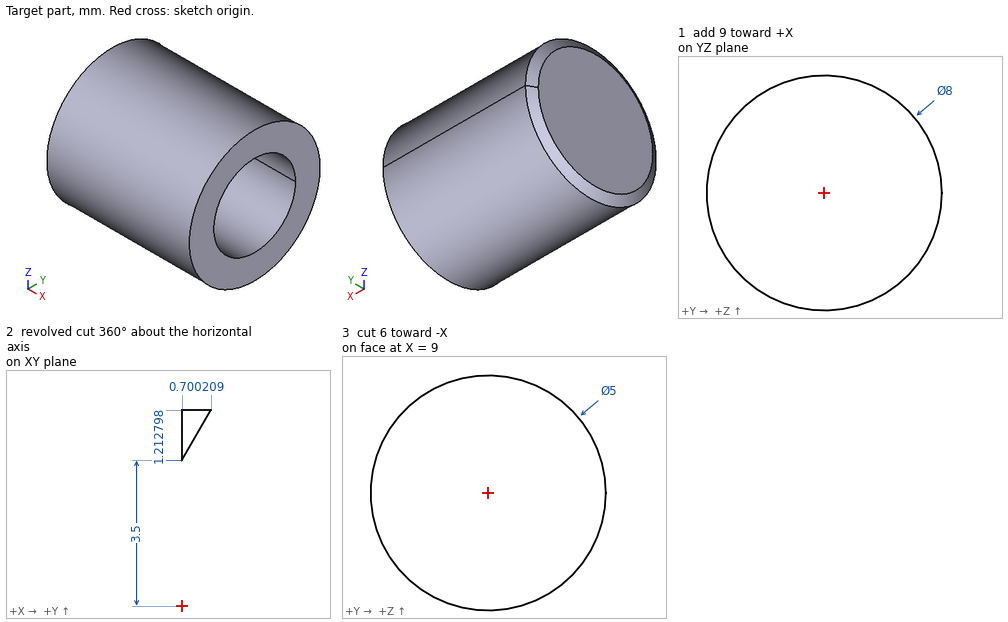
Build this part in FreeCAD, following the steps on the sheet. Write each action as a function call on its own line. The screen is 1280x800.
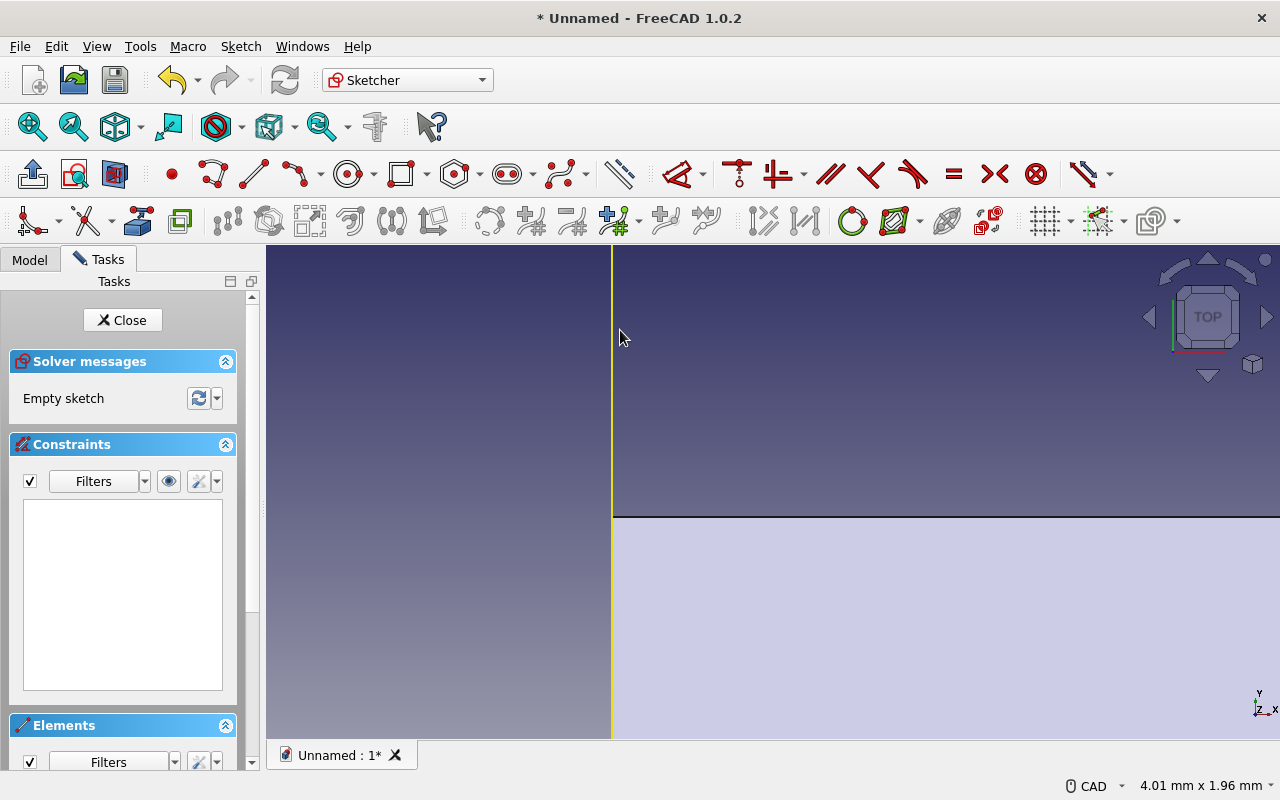
click(213, 174)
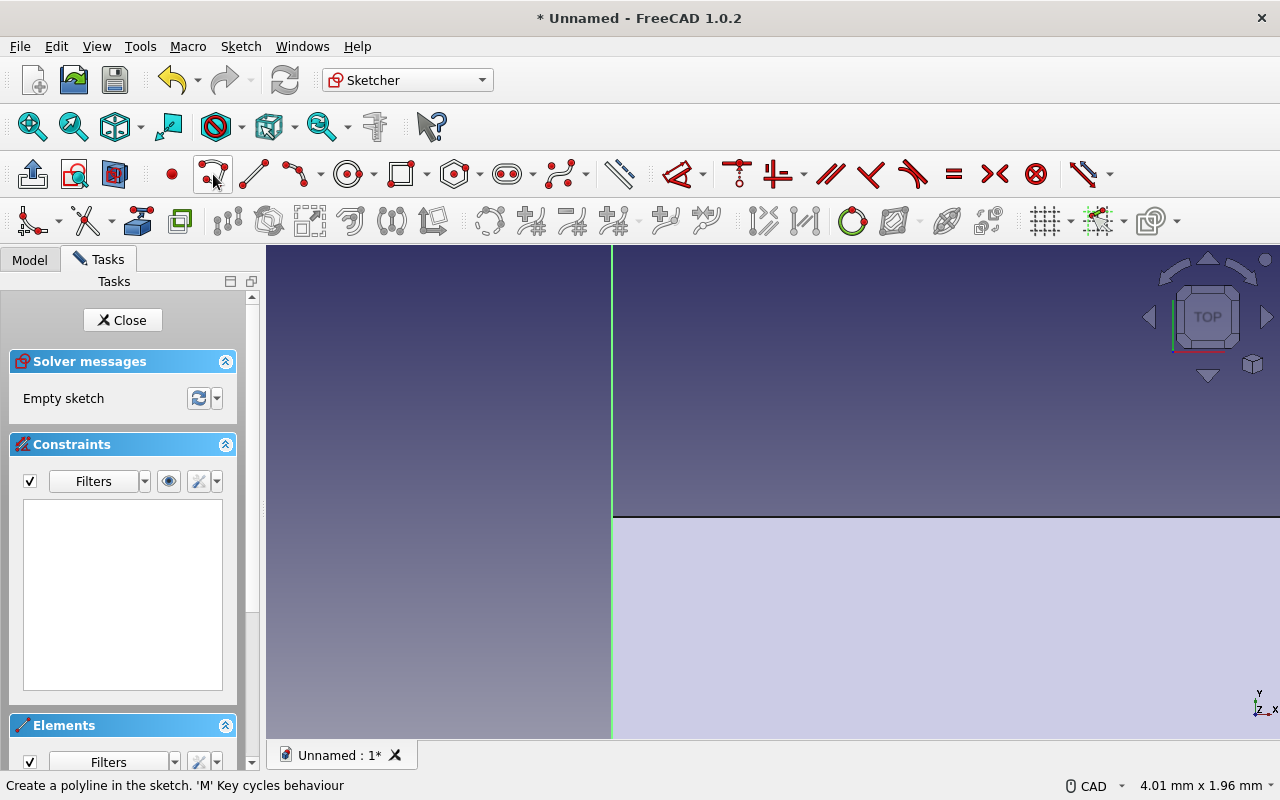
click(612, 643)
click(788, 336)
click(621, 336)
click(612, 644)
key(Escape)
key(Escape)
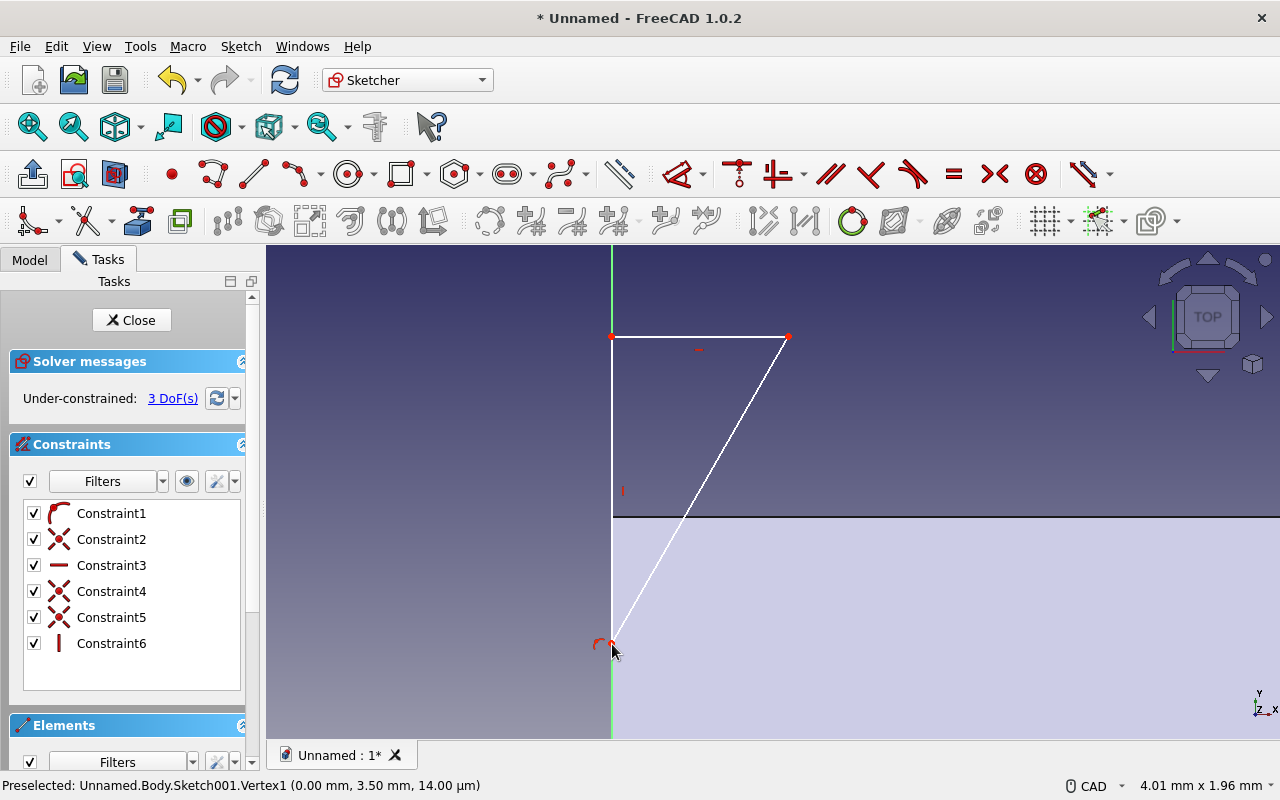
click(676, 174)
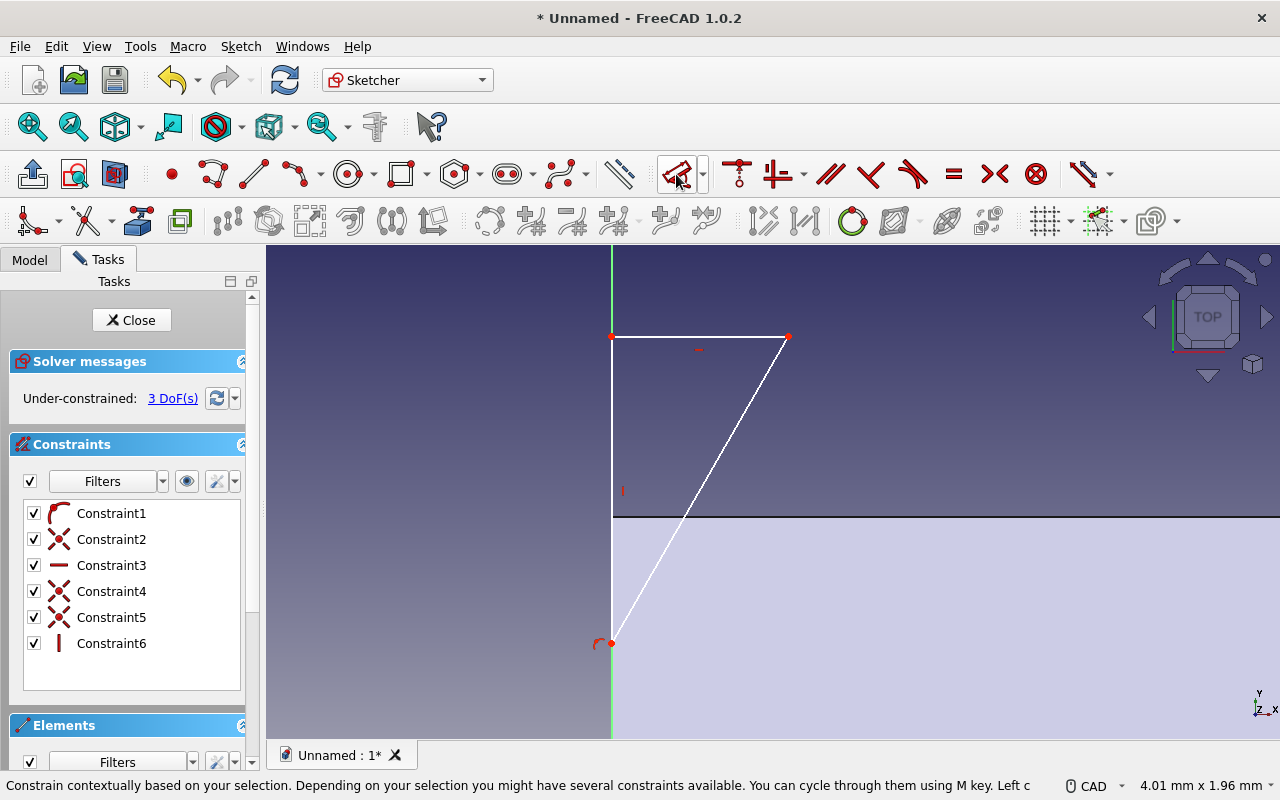
click(612, 644)
click(578, 677)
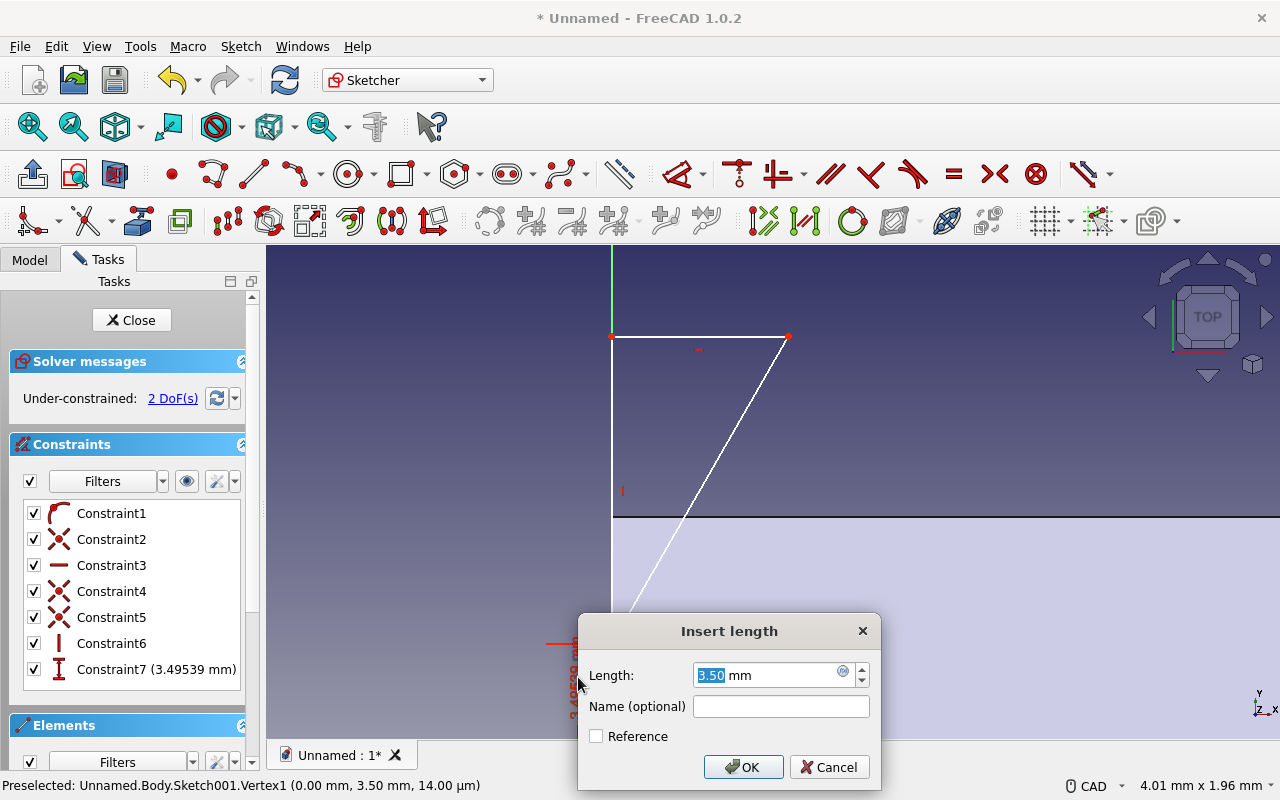
text(3.5)
key(Return)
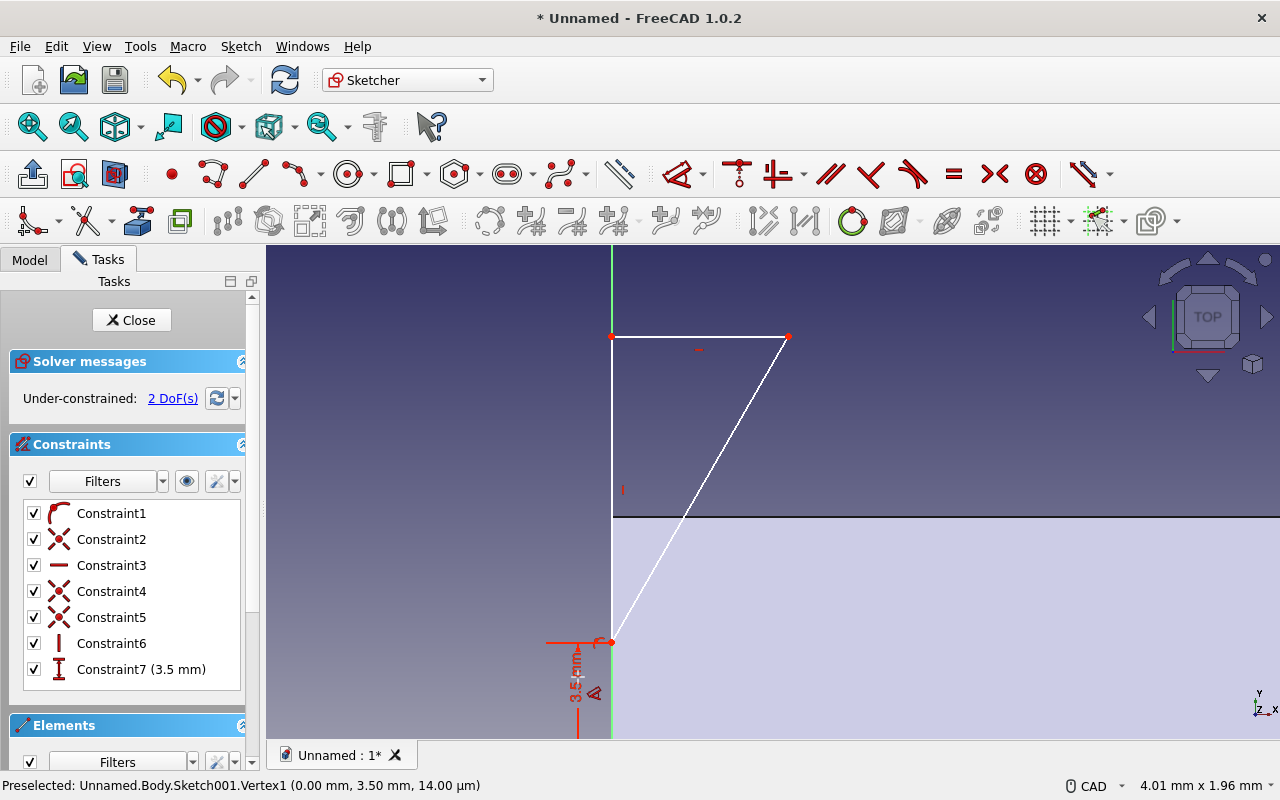
click(735, 337)
click(700, 303)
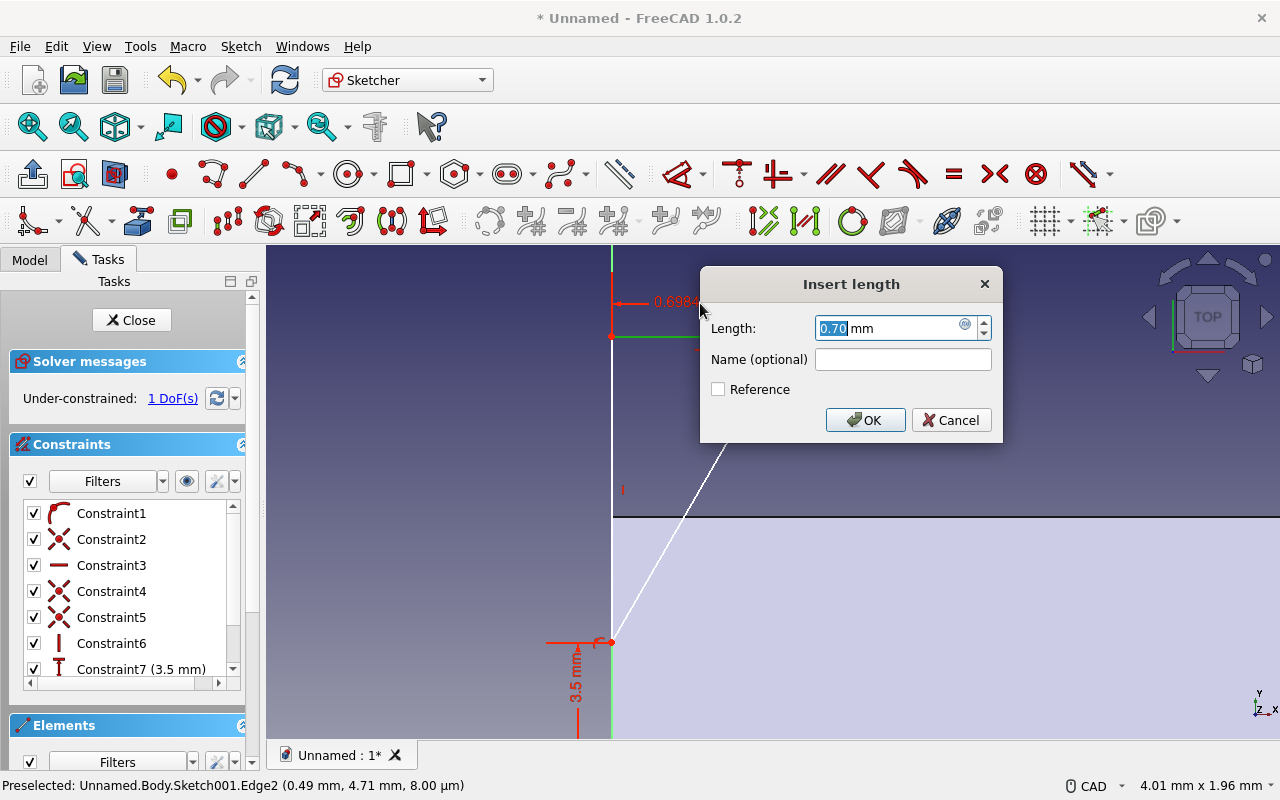
text(0.700209)
key(Return)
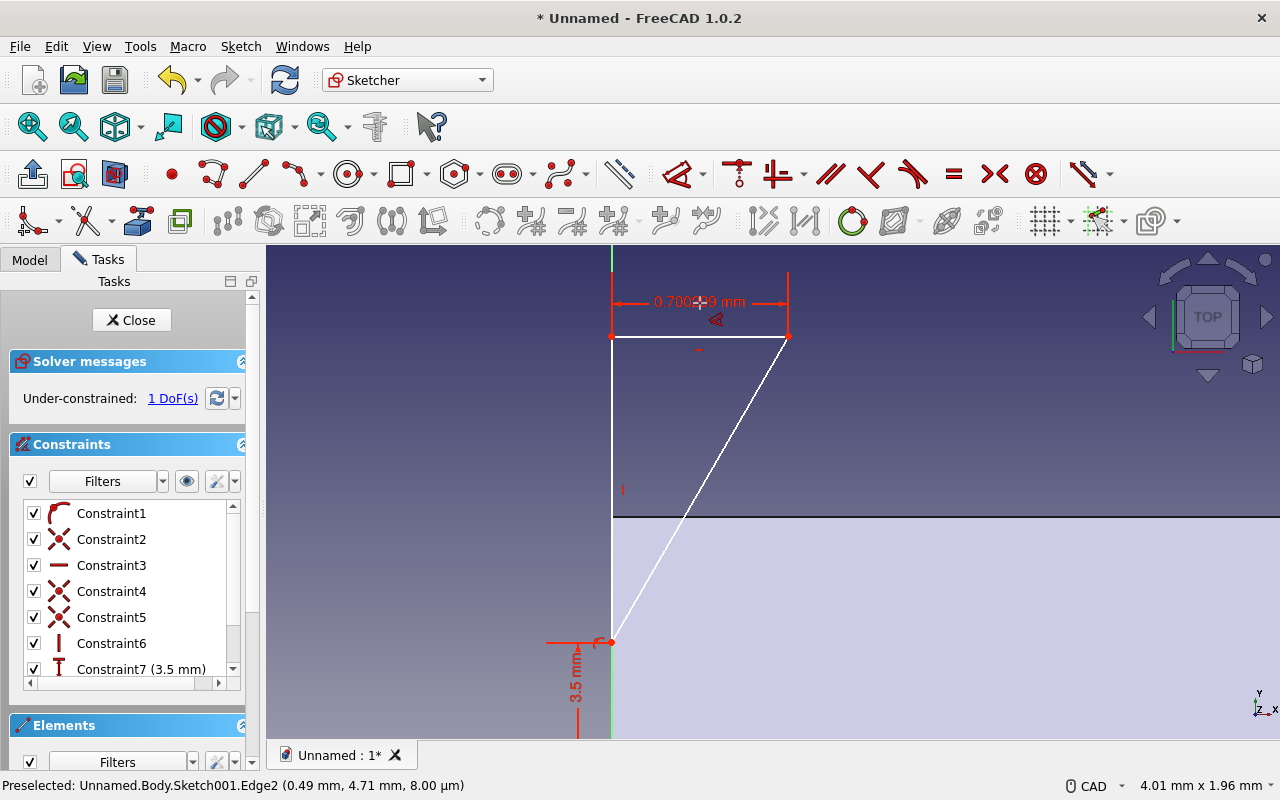
click(612, 429)
click(578, 490)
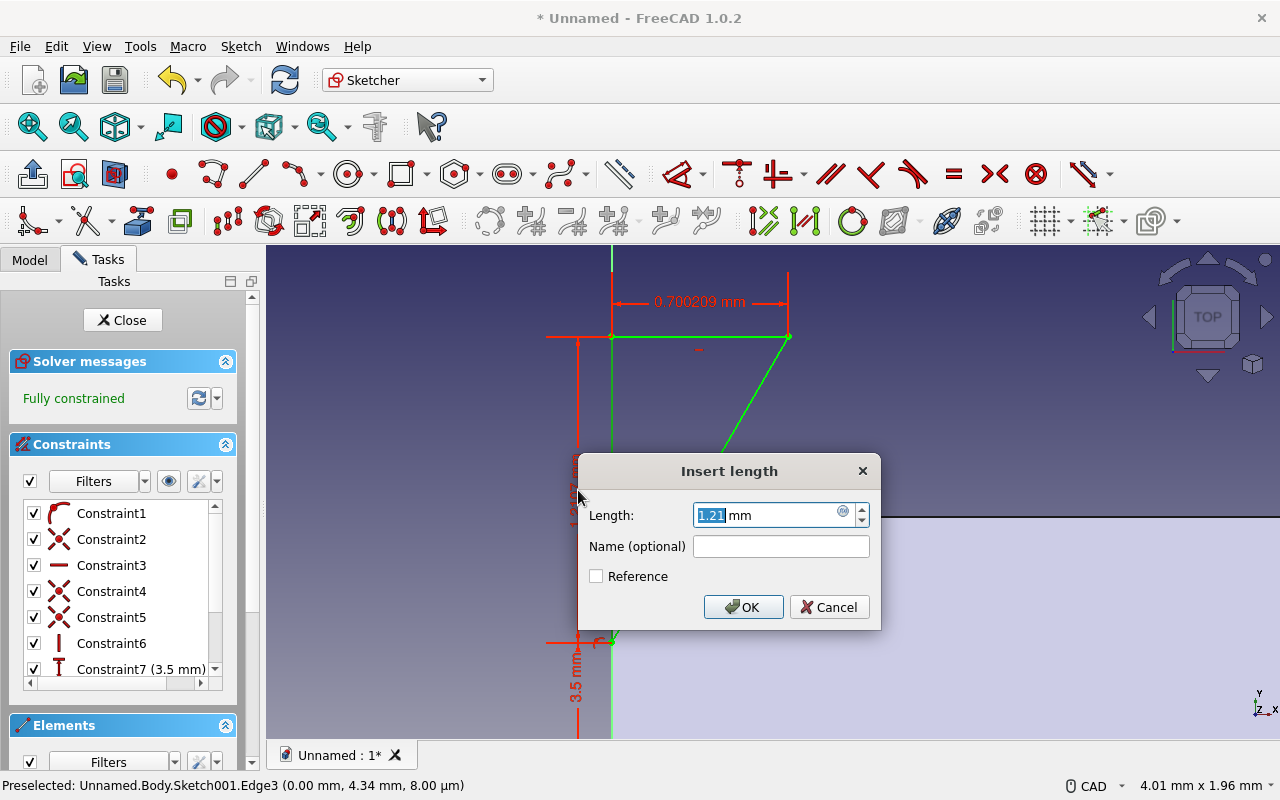
text(1.212798)
key(Return)
key(Escape)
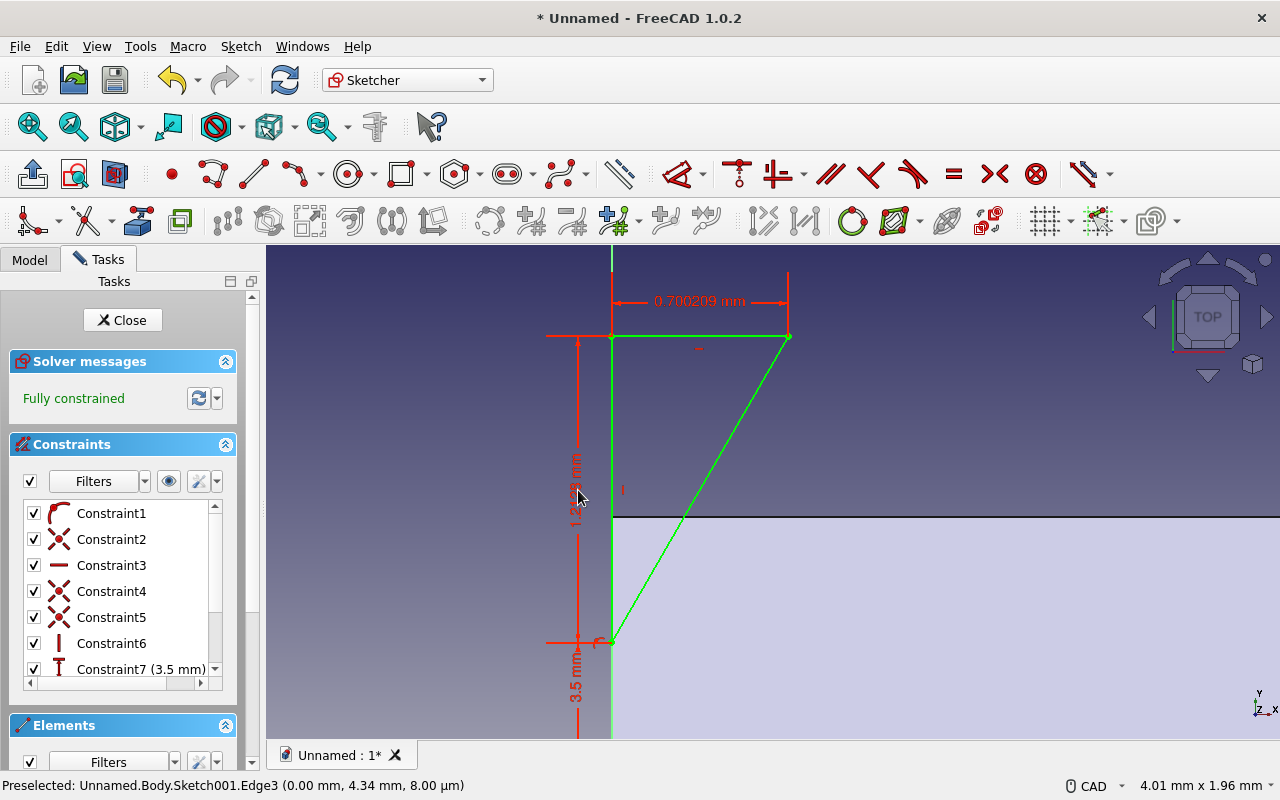
click(123, 320)